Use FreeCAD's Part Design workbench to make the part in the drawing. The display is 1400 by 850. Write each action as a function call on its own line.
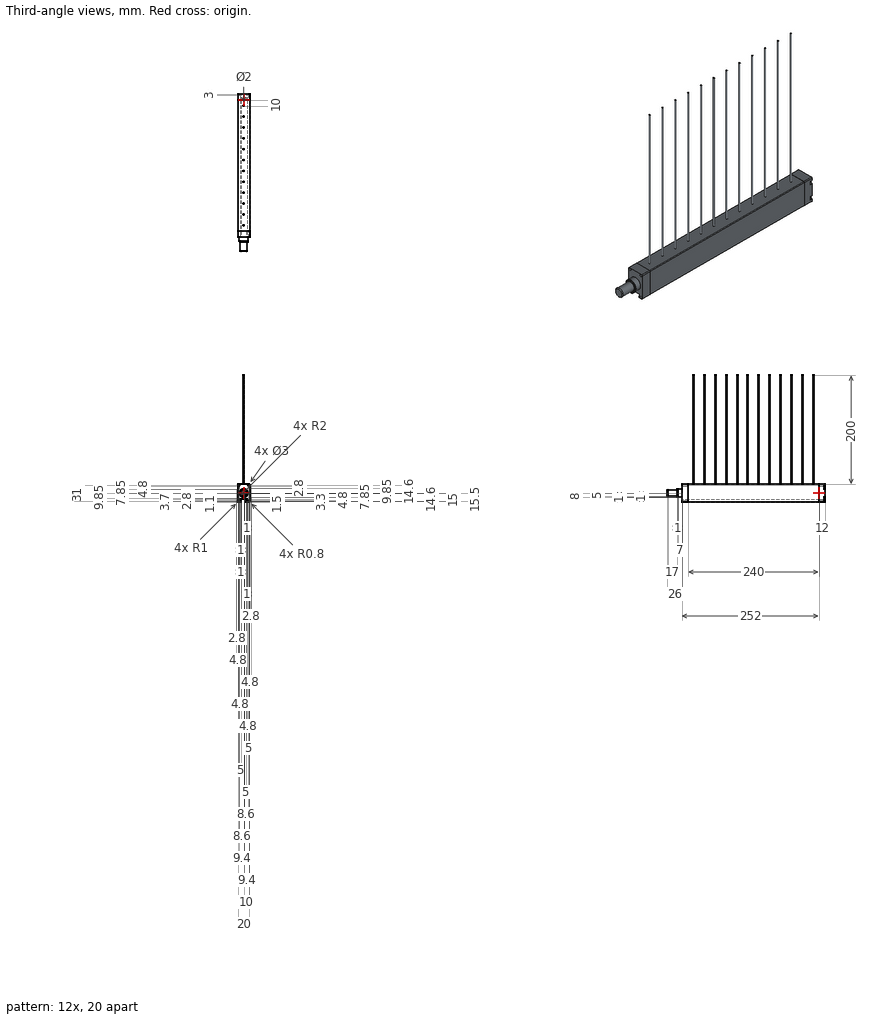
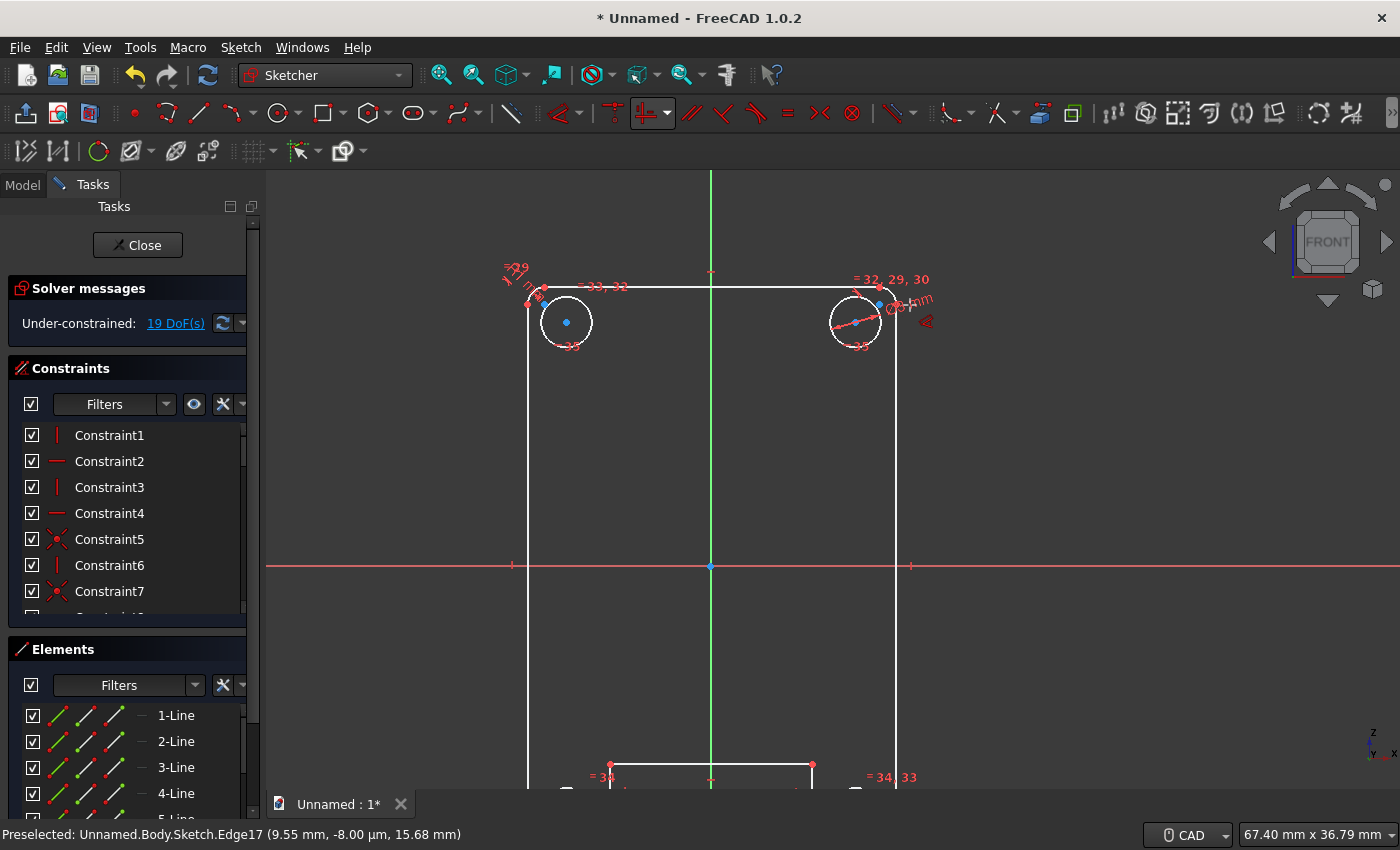
scroll(873, 303, down, 2)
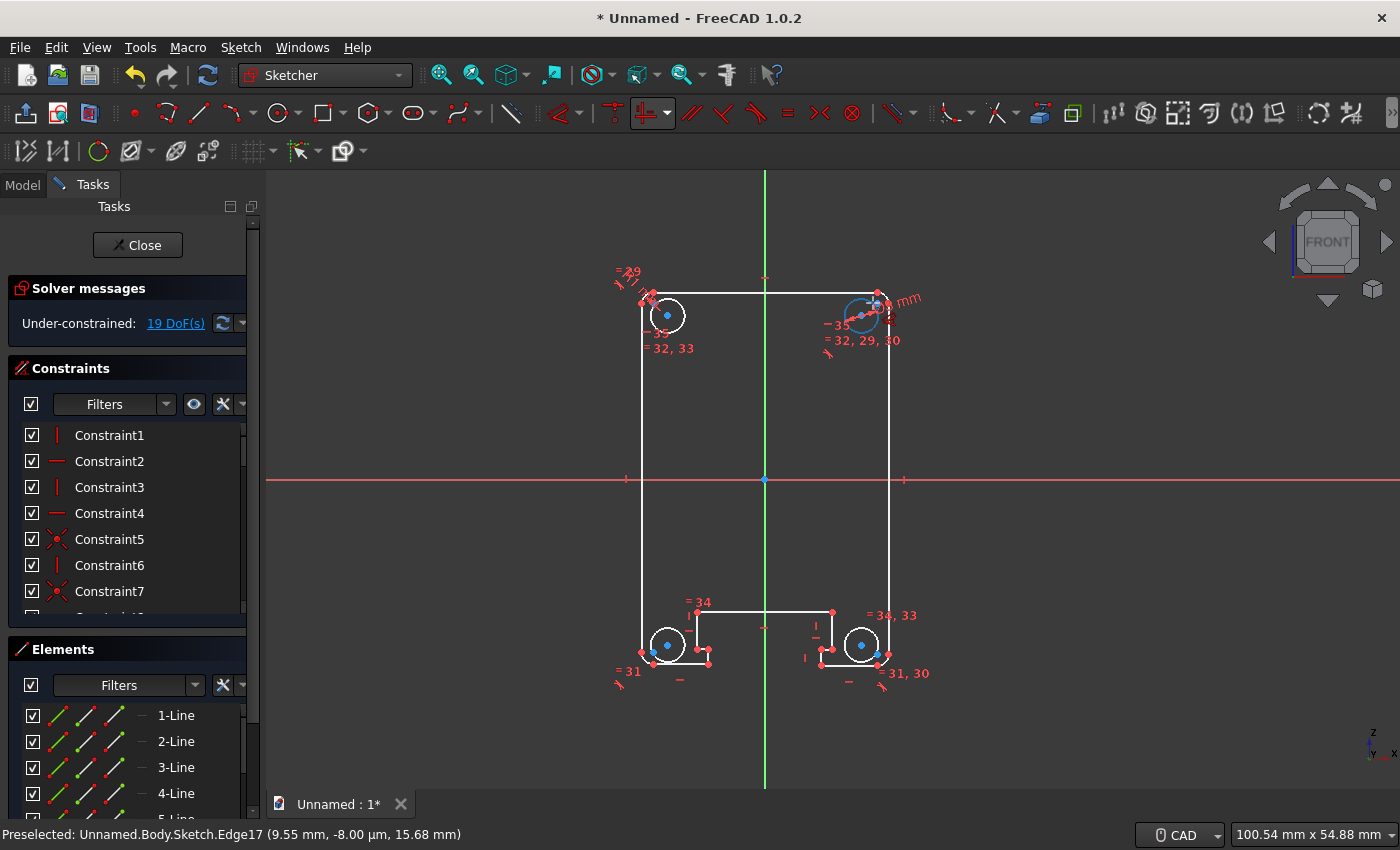
click(838, 666)
click(849, 700)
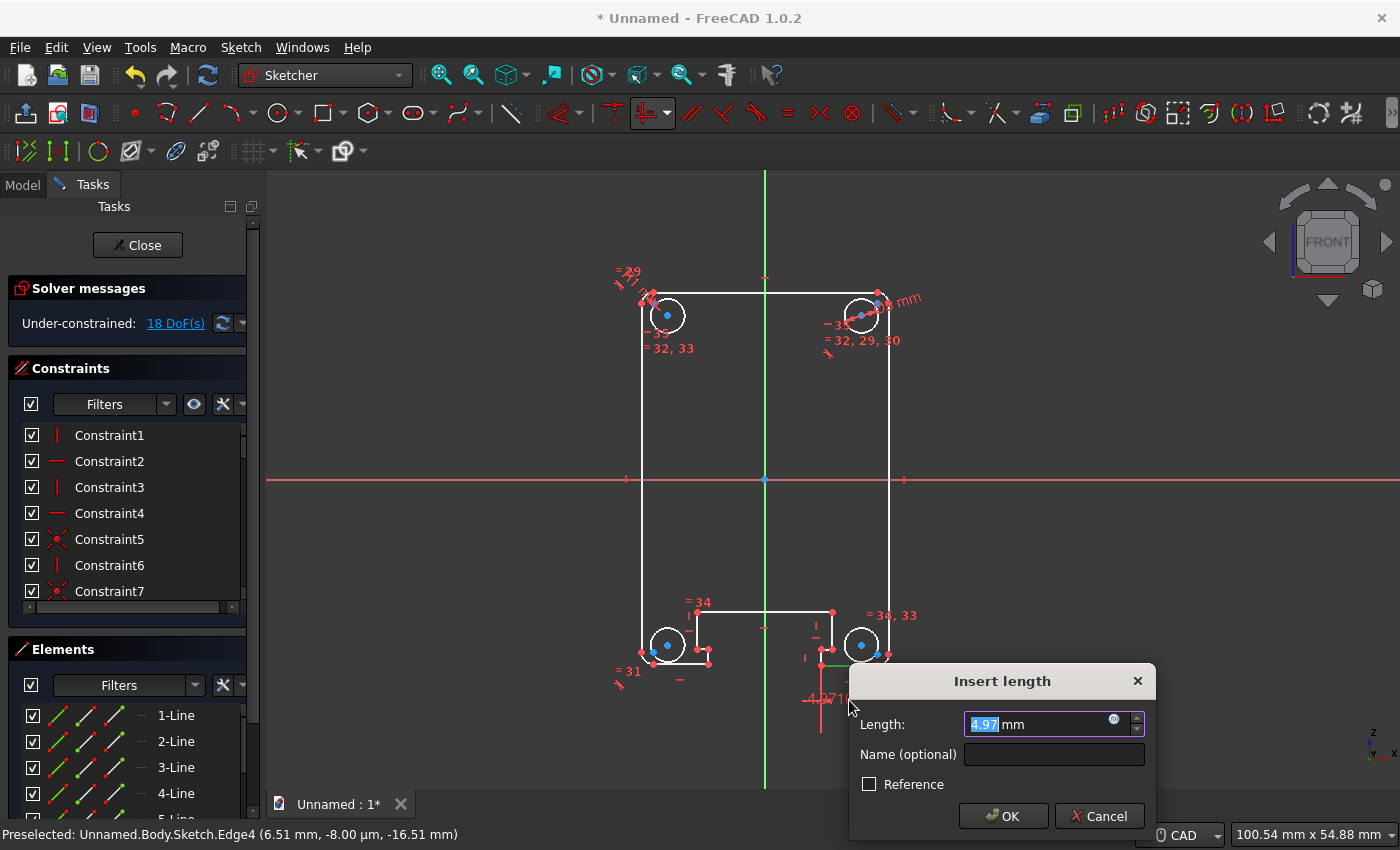
text(5)
key(Return)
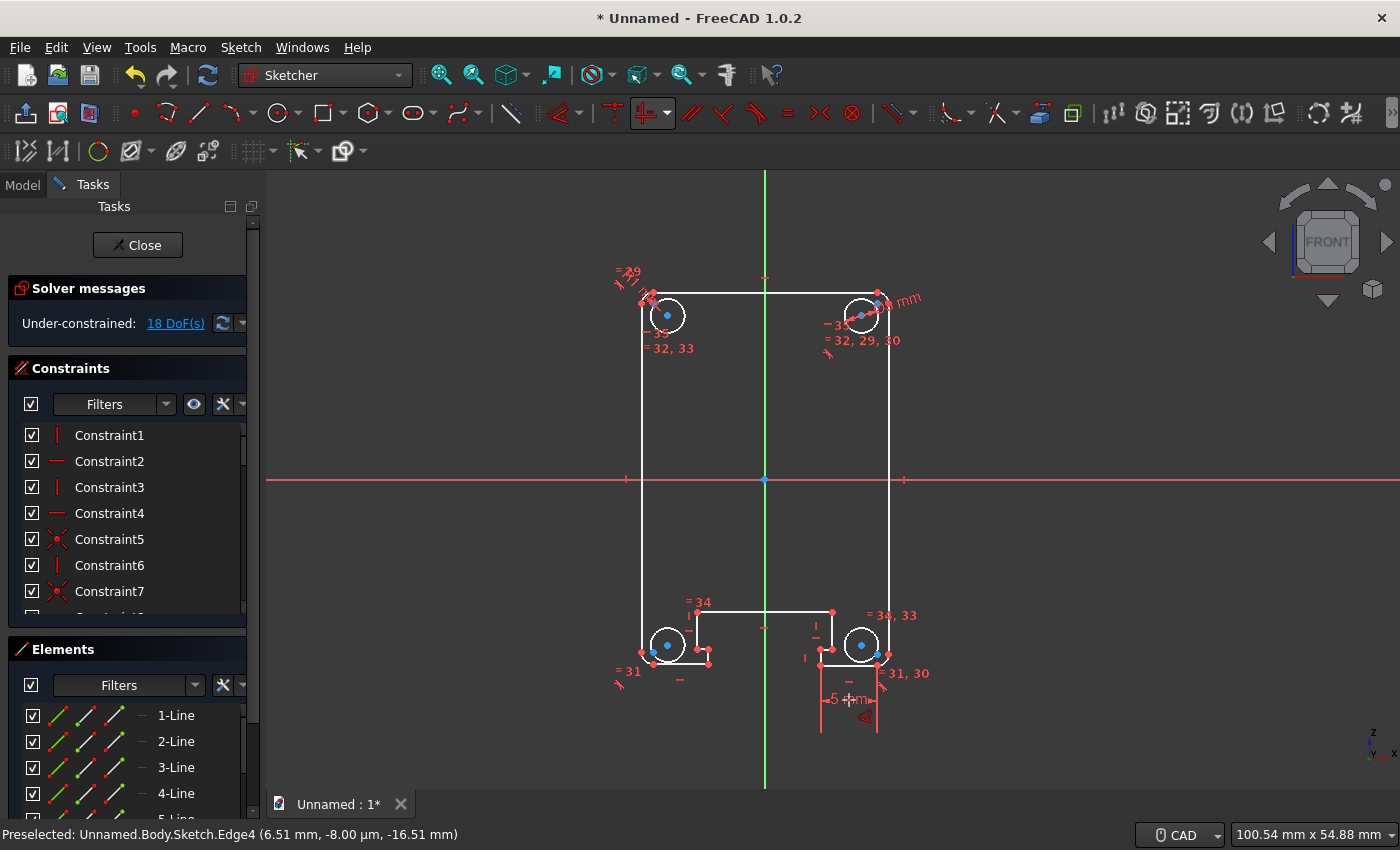
scroll(827, 650, up, 7)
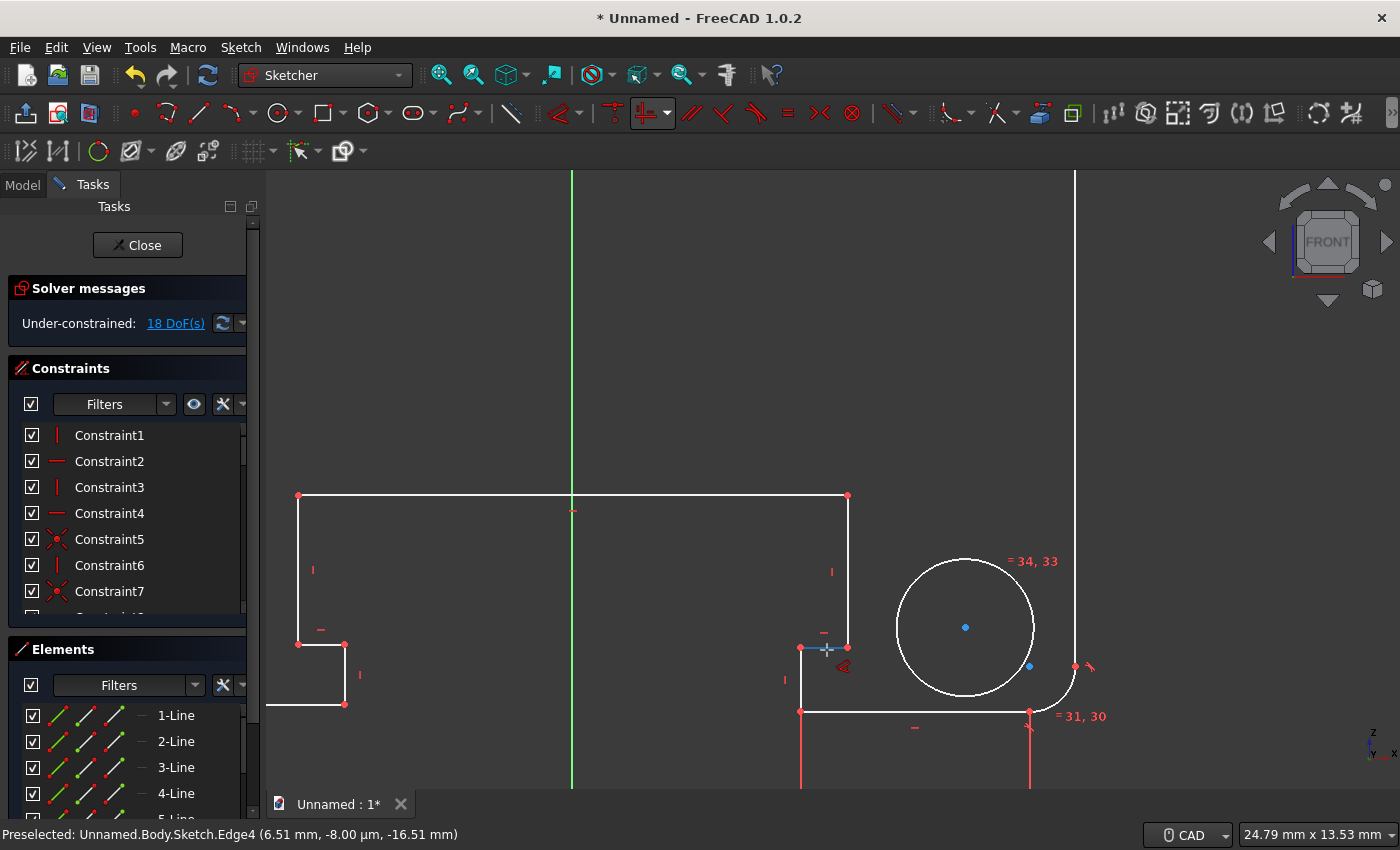
click(824, 648)
click(824, 682)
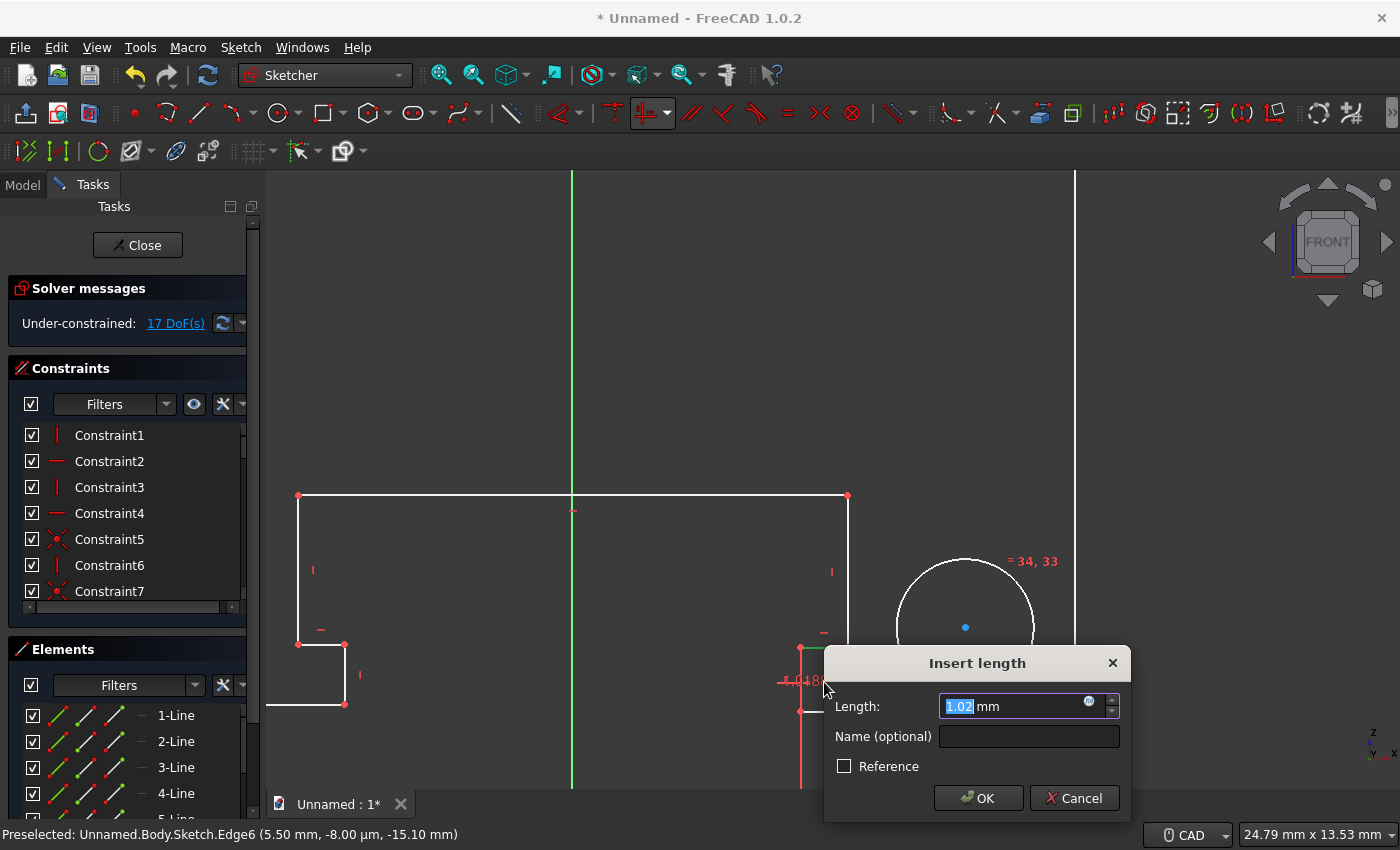
text(1)
key(Return)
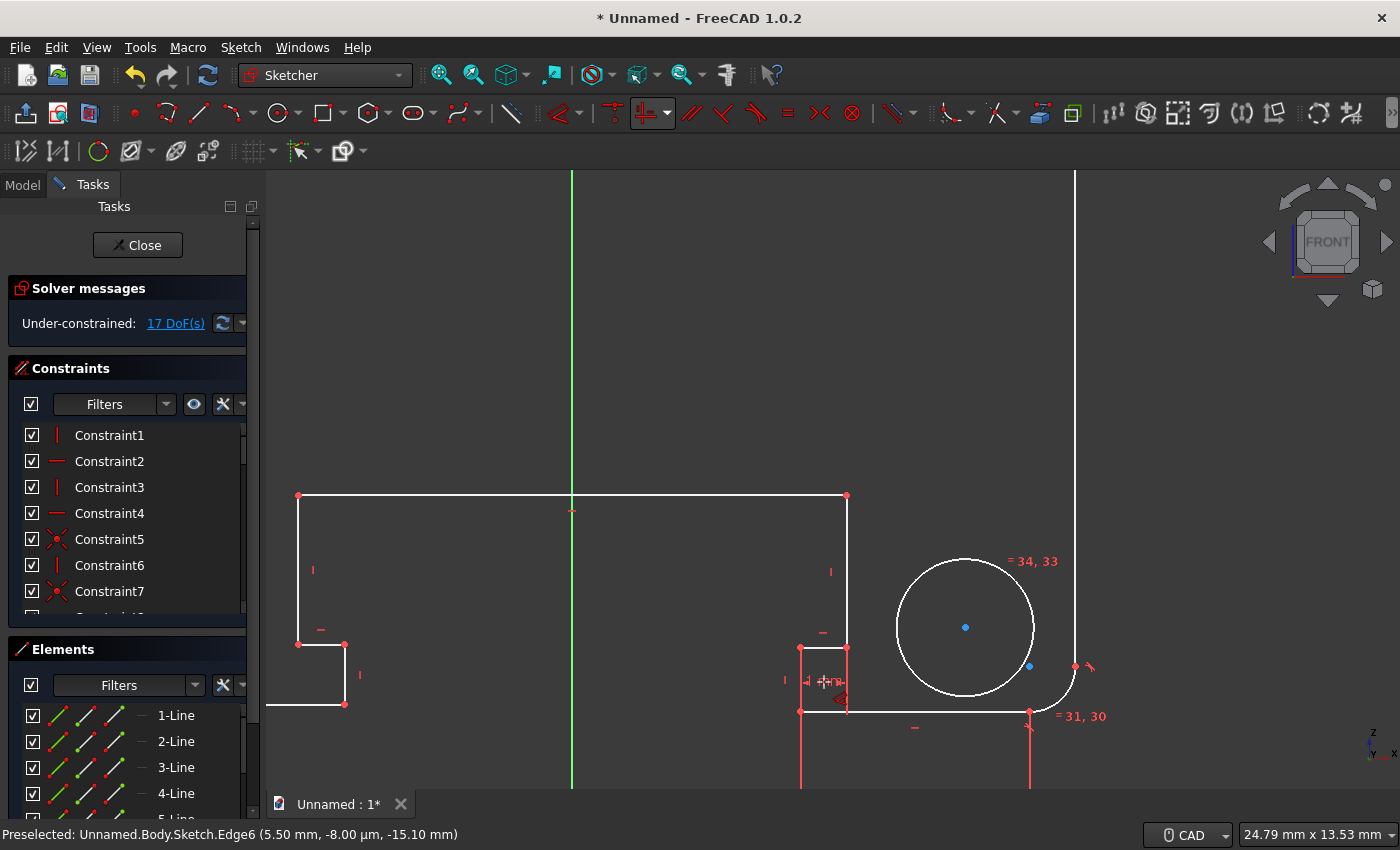
click(312, 645)
click(322, 679)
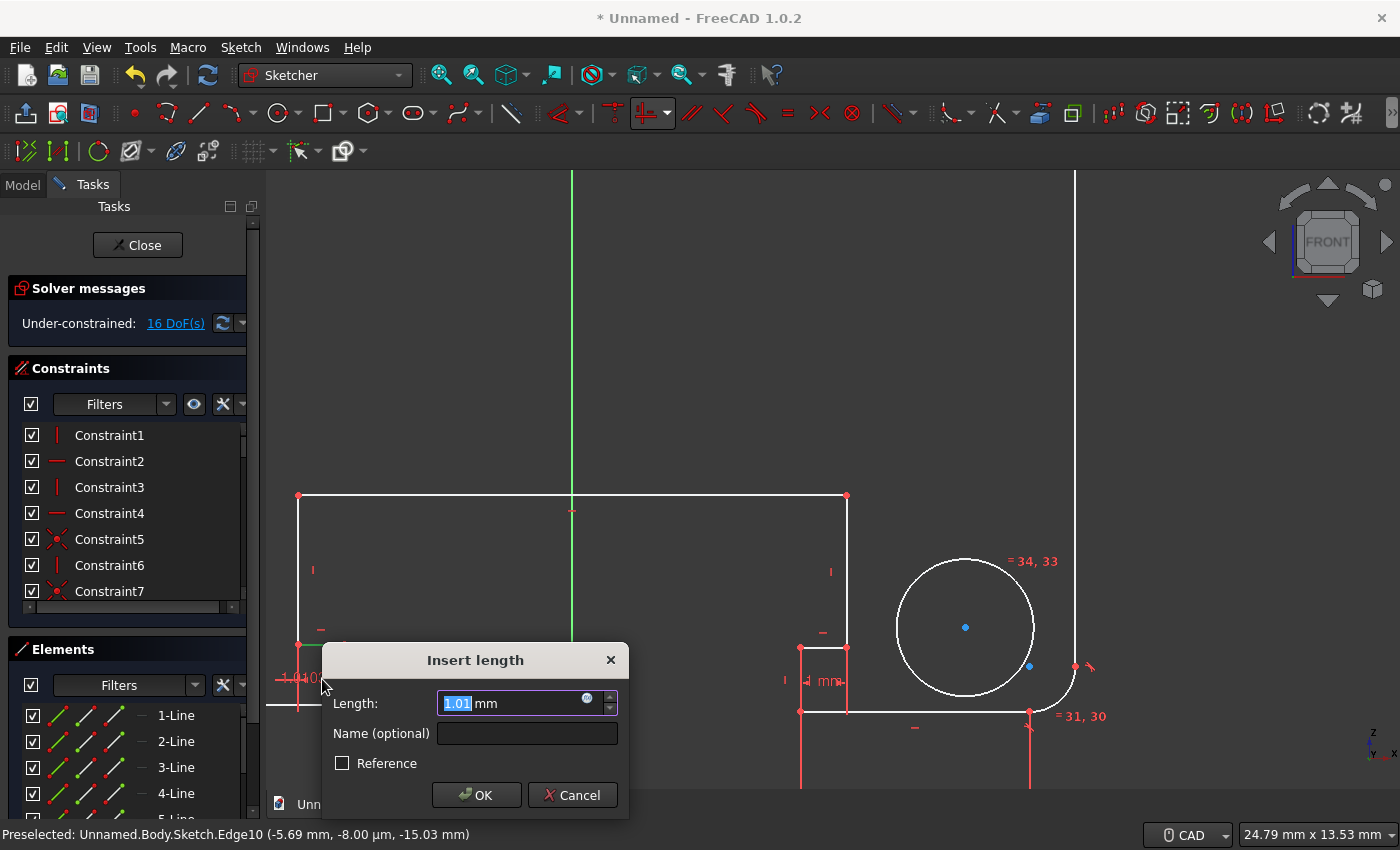
text(1)
key(Return)